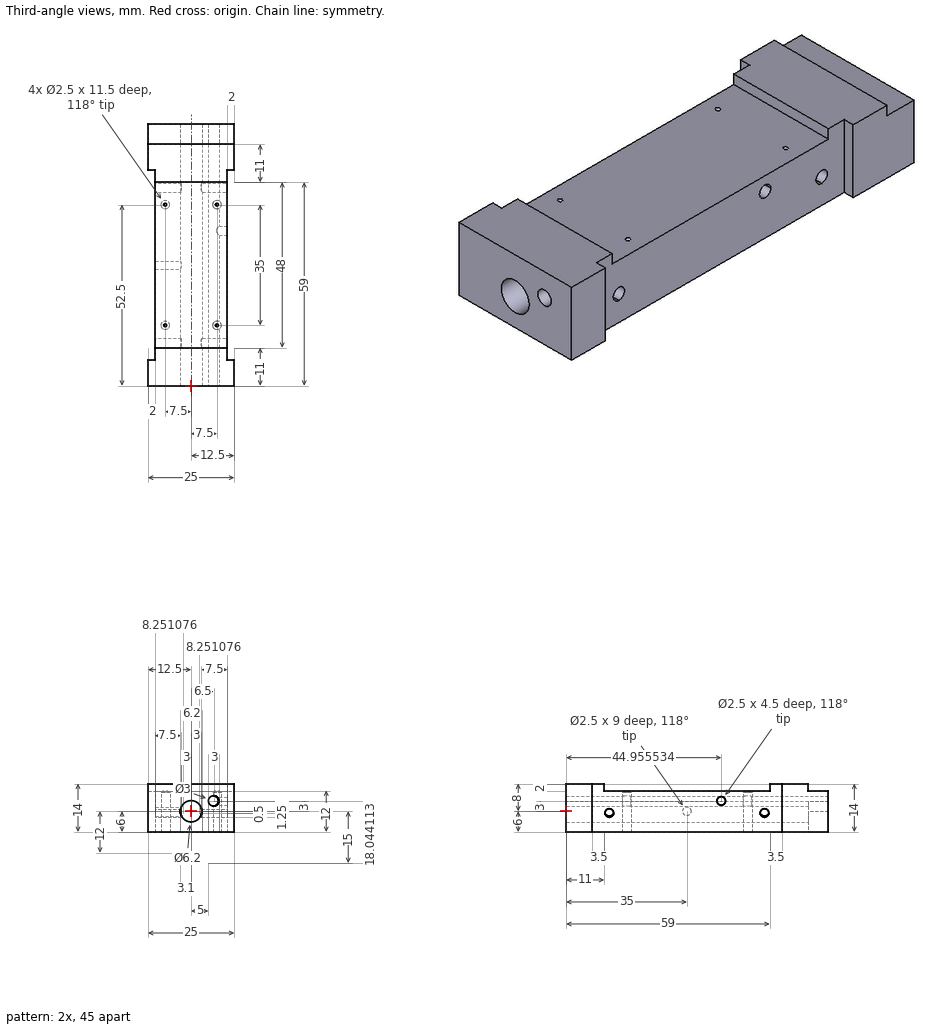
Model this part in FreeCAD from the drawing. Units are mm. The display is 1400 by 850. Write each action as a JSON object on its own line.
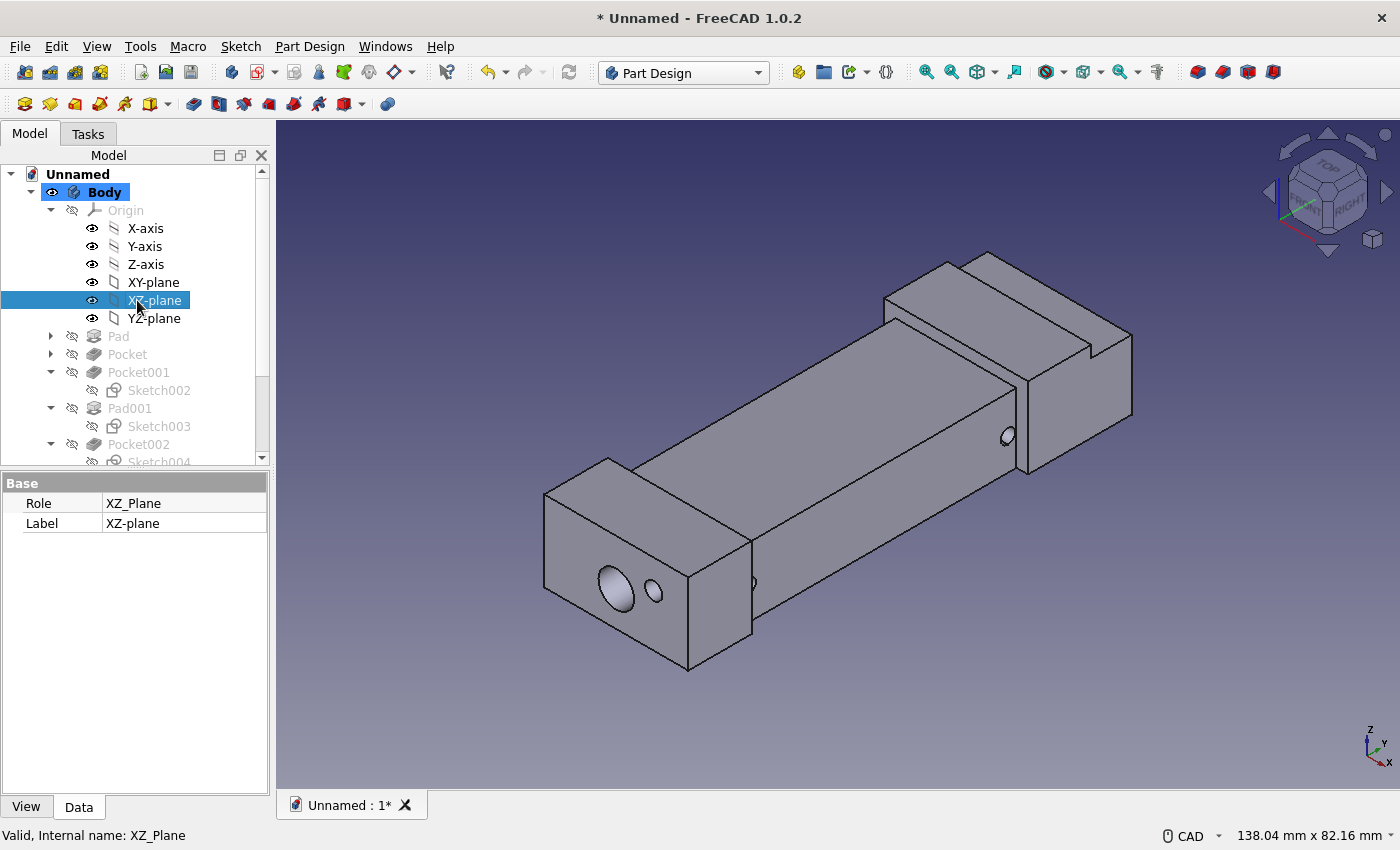
{"action": "left_click", "coordinate": [394, 72]}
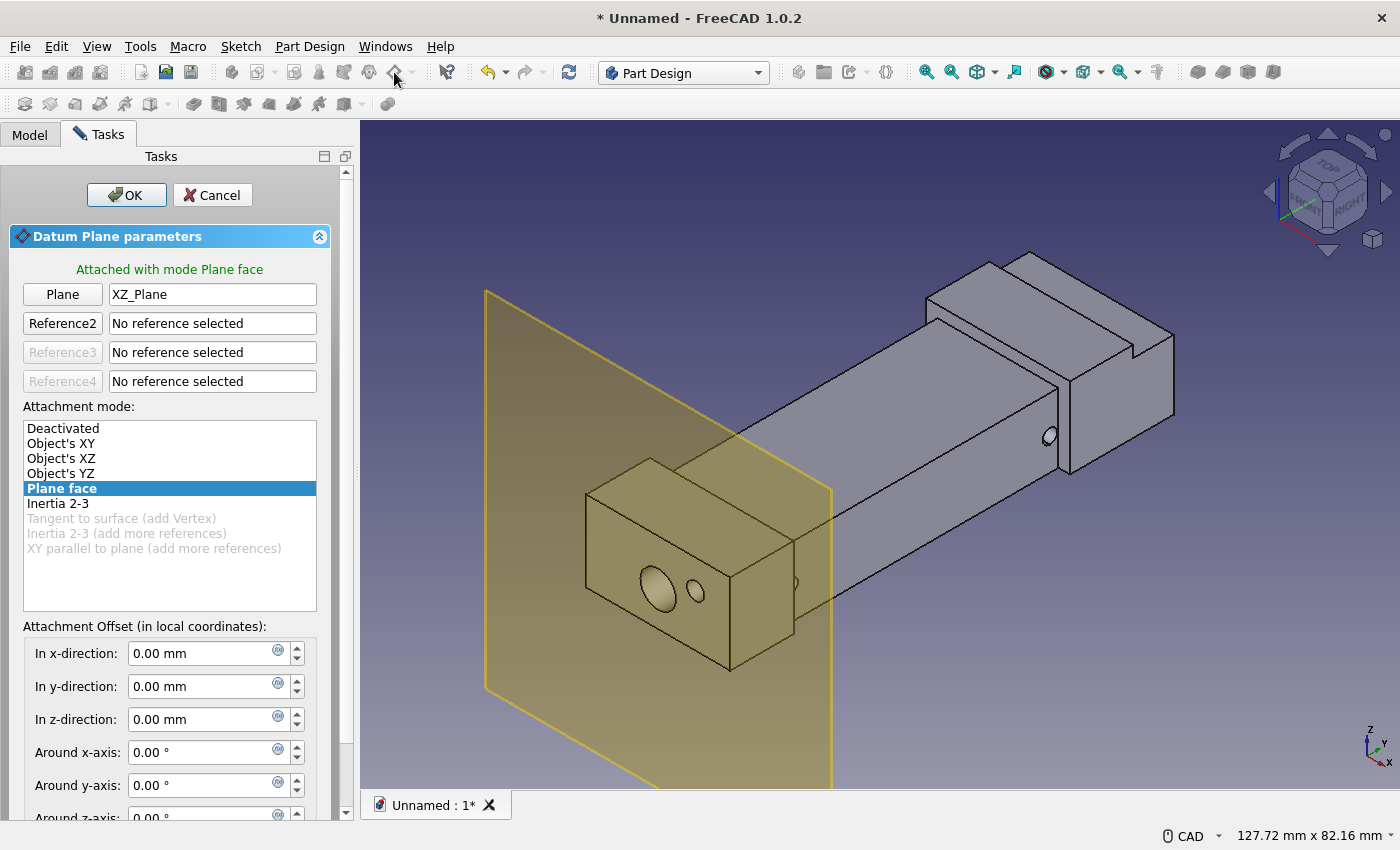
{"action": "triple_click", "coordinate": [210, 720]}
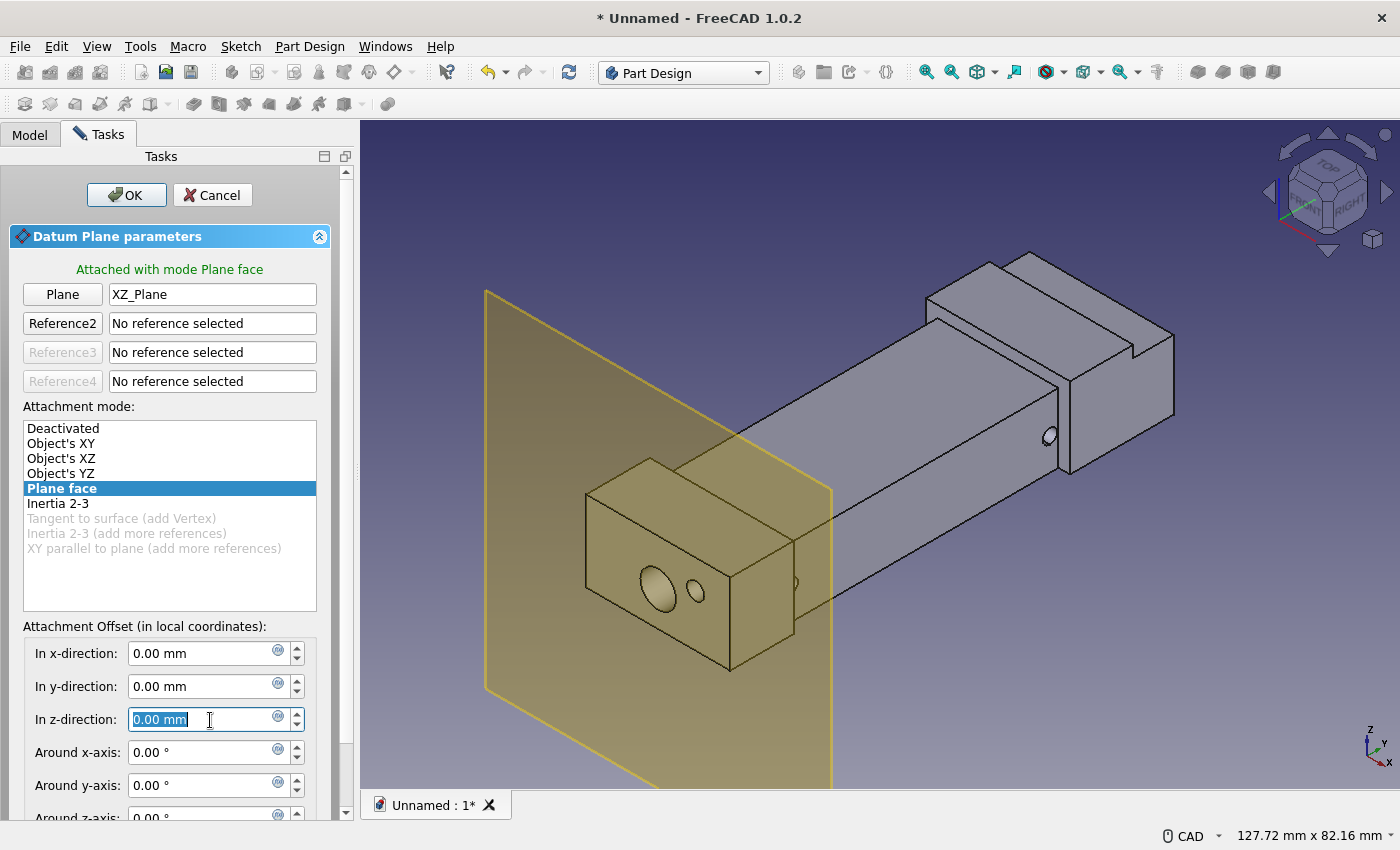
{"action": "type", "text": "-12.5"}
{"action": "key", "text": "Tab"}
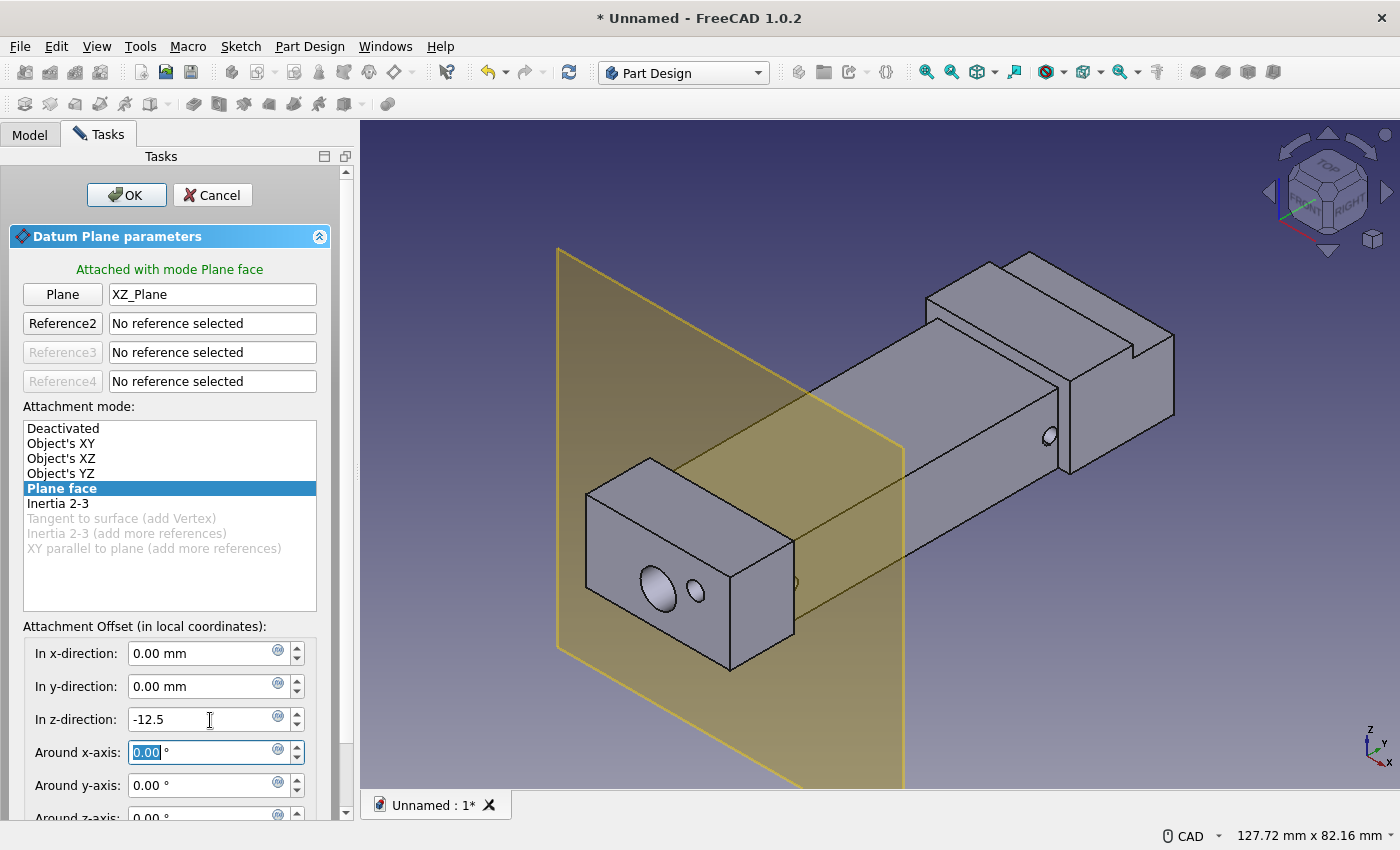
{"action": "left_click", "coordinate": [127, 195]}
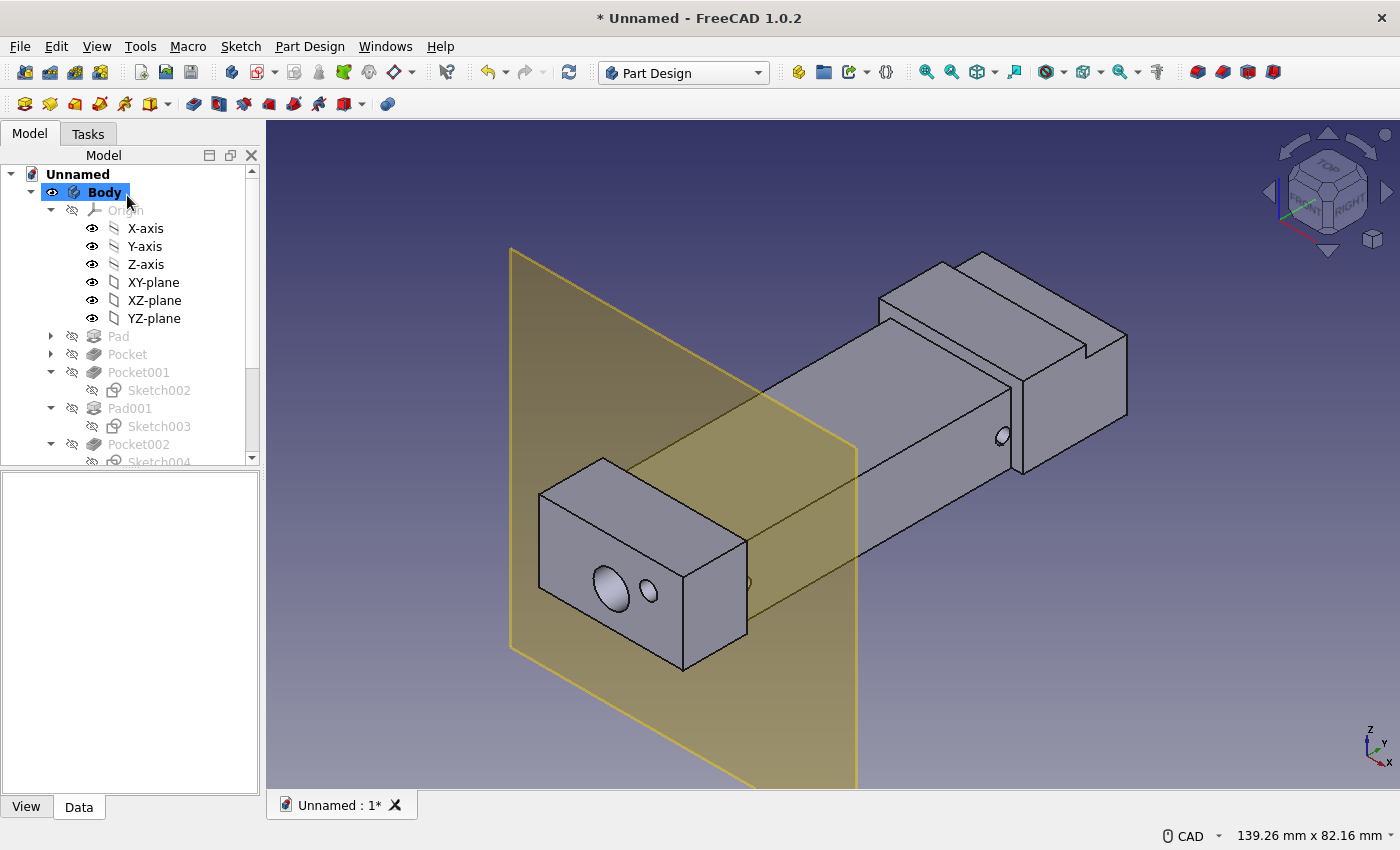
{"action": "scroll", "coordinate": [101, 314], "scroll_direction": "down", "scroll_amount": 3}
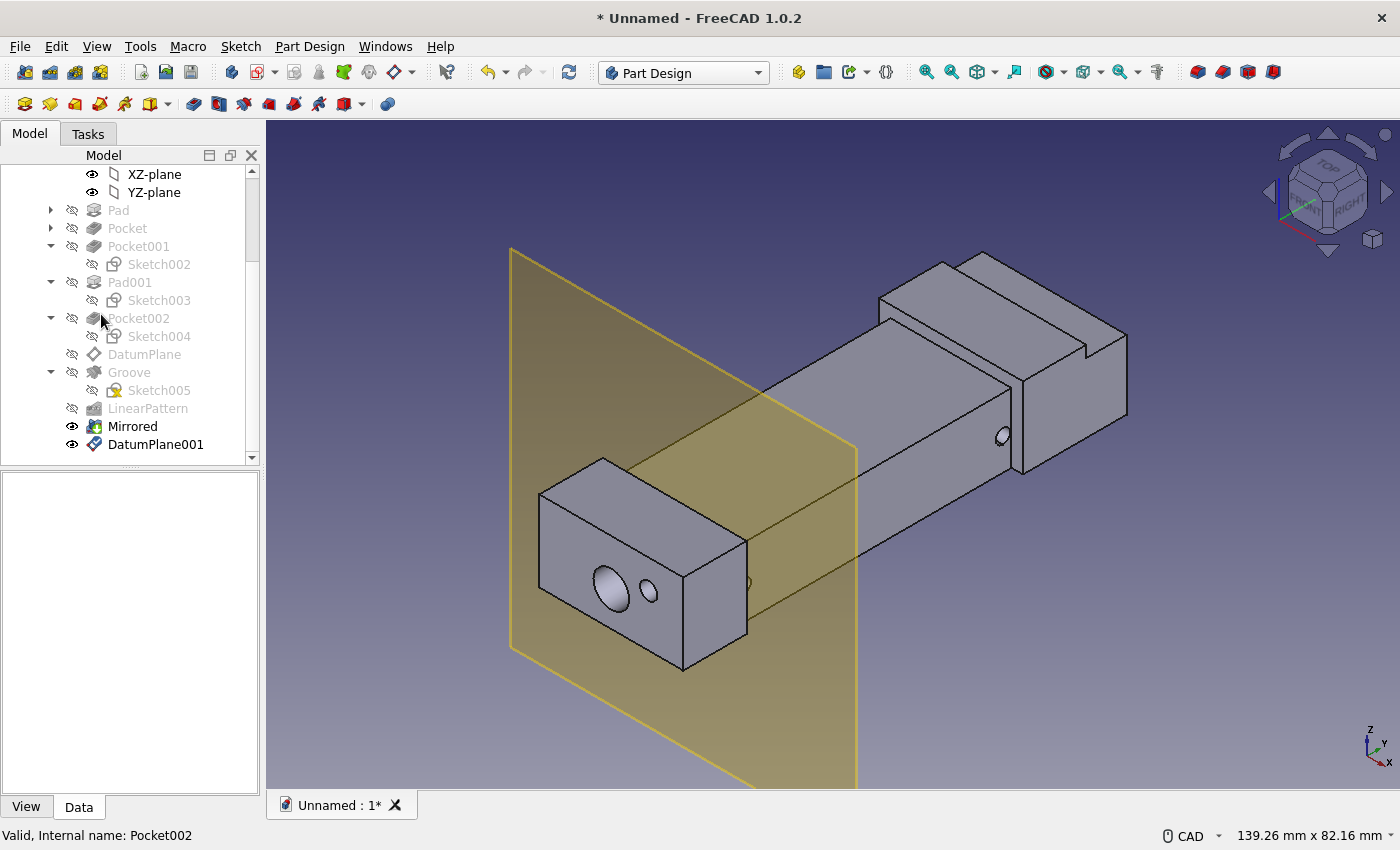
{"action": "left_click", "coordinate": [117, 444]}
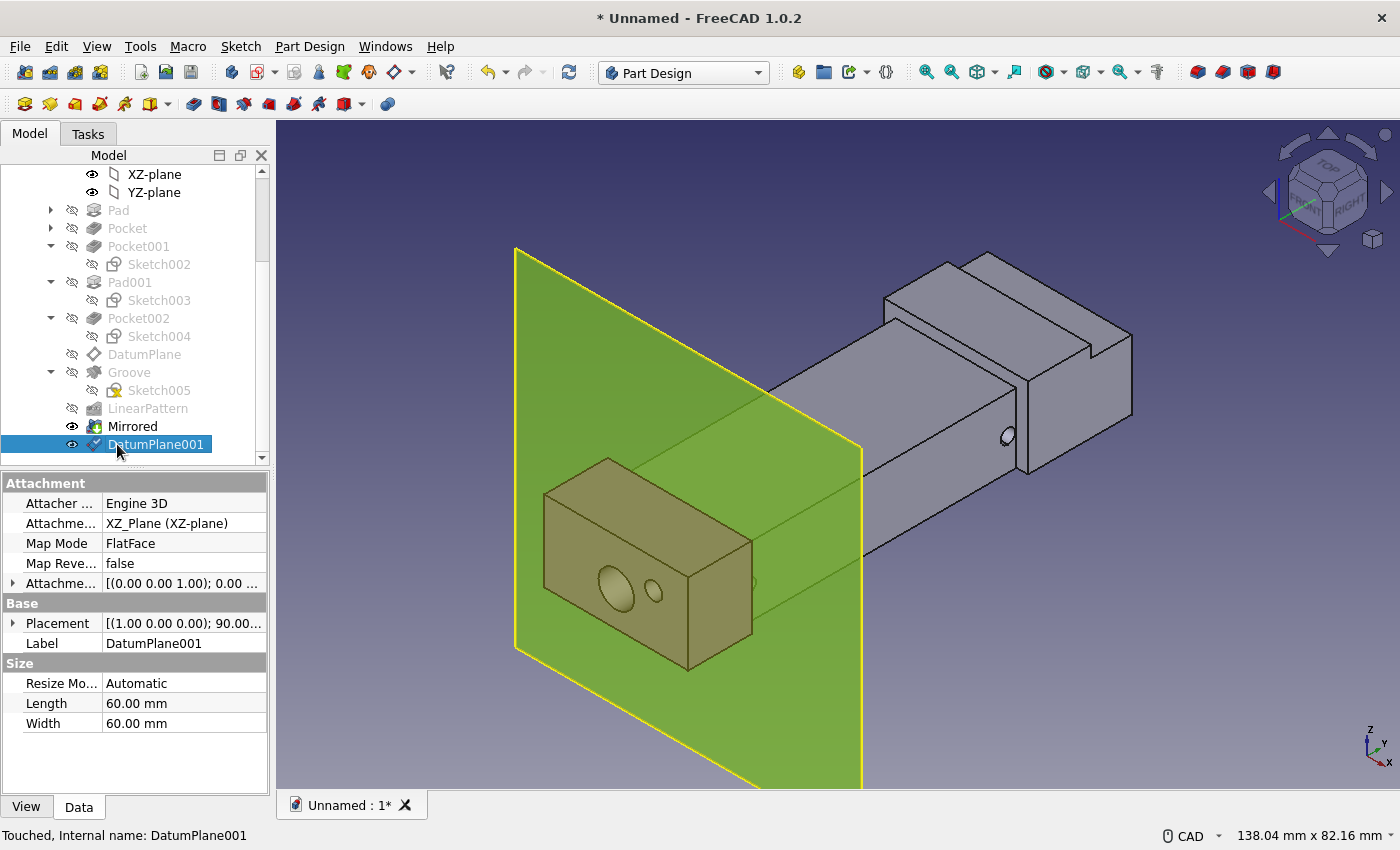
{"action": "left_click", "coordinate": [256, 72]}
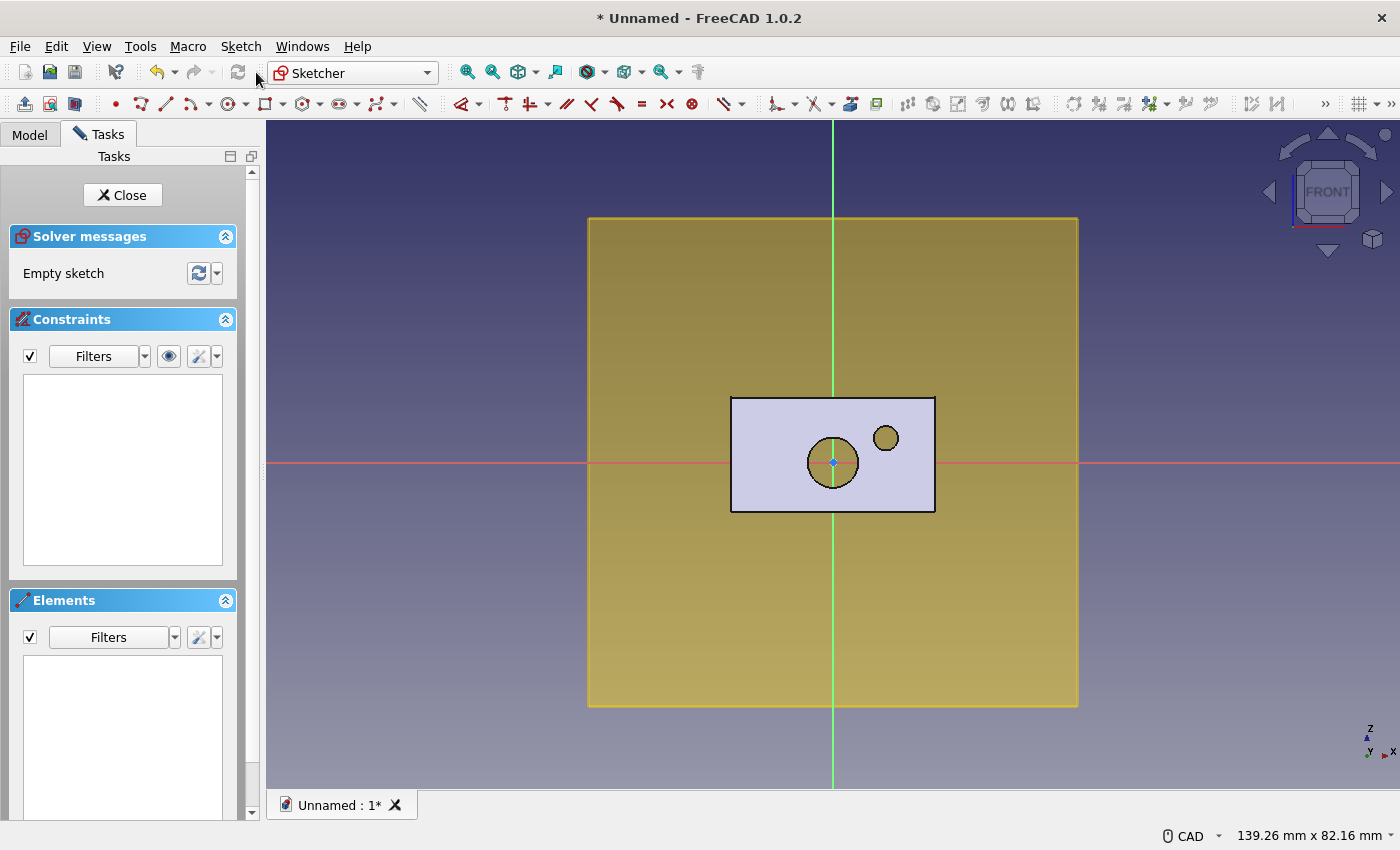
{"action": "left_click", "coordinate": [75, 104]}